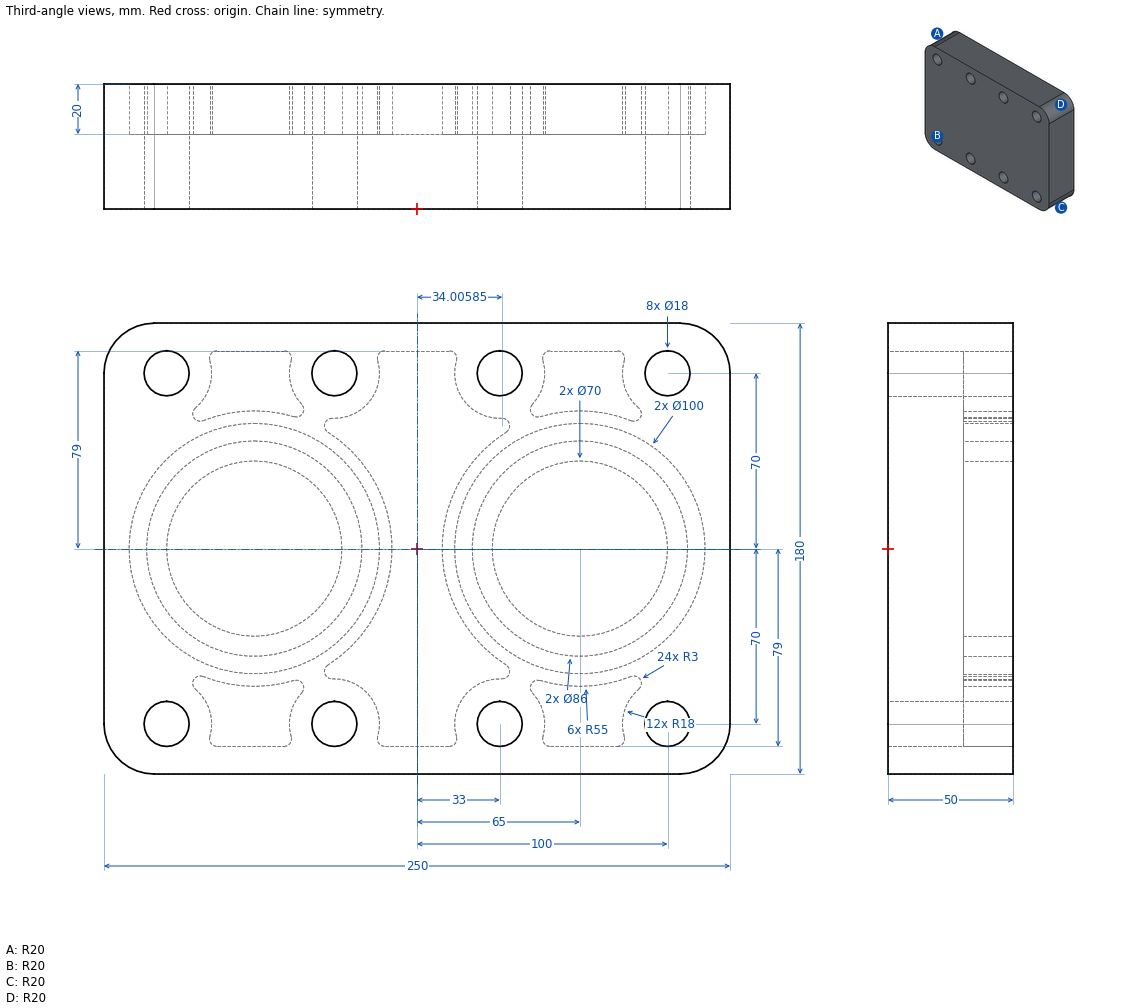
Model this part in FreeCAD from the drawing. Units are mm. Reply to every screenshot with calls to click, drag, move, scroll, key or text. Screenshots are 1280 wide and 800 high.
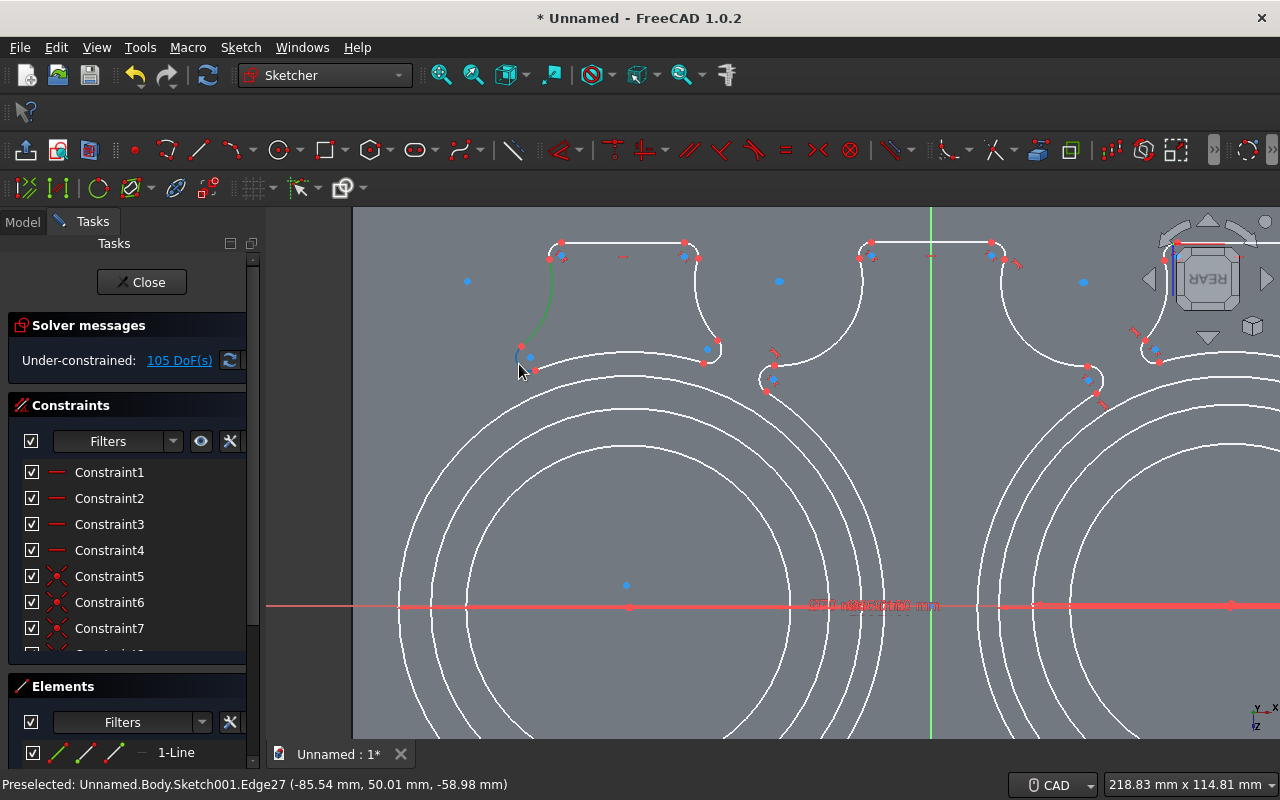
click(518, 365)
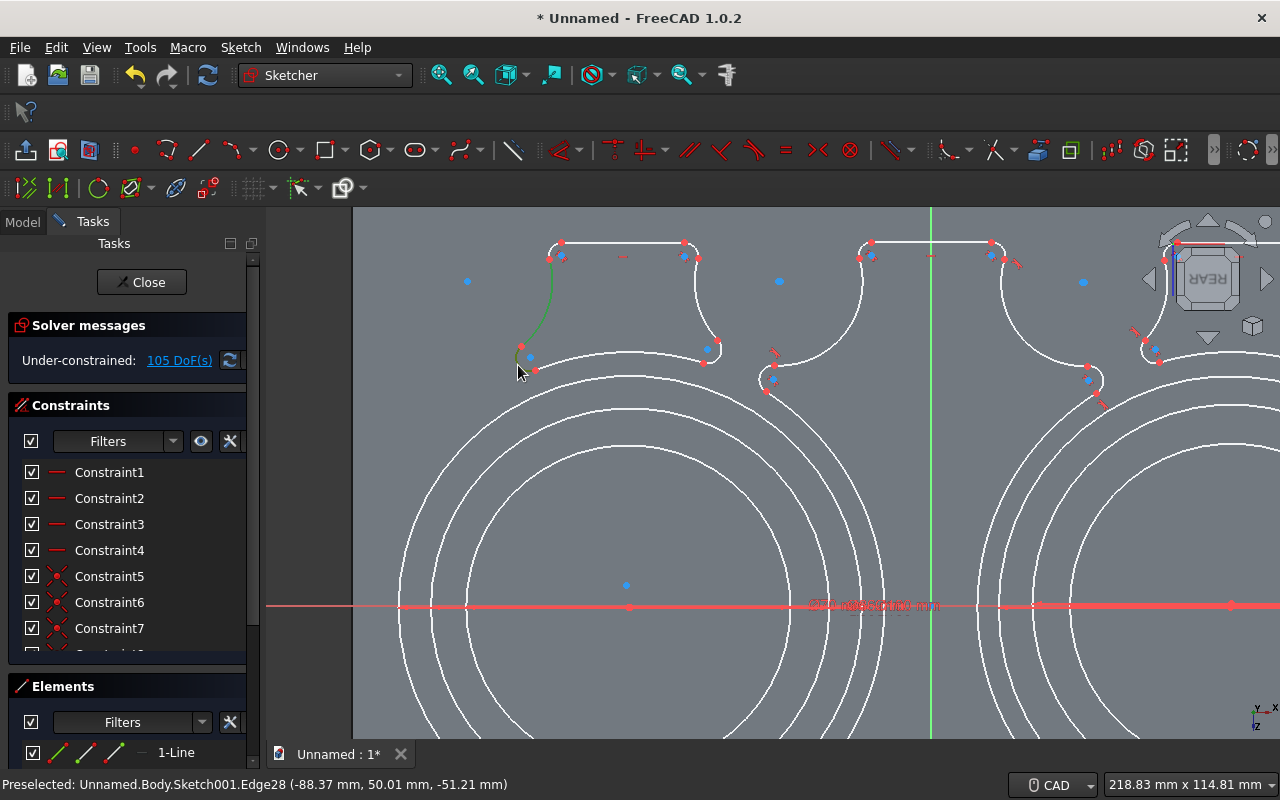
click(754, 150)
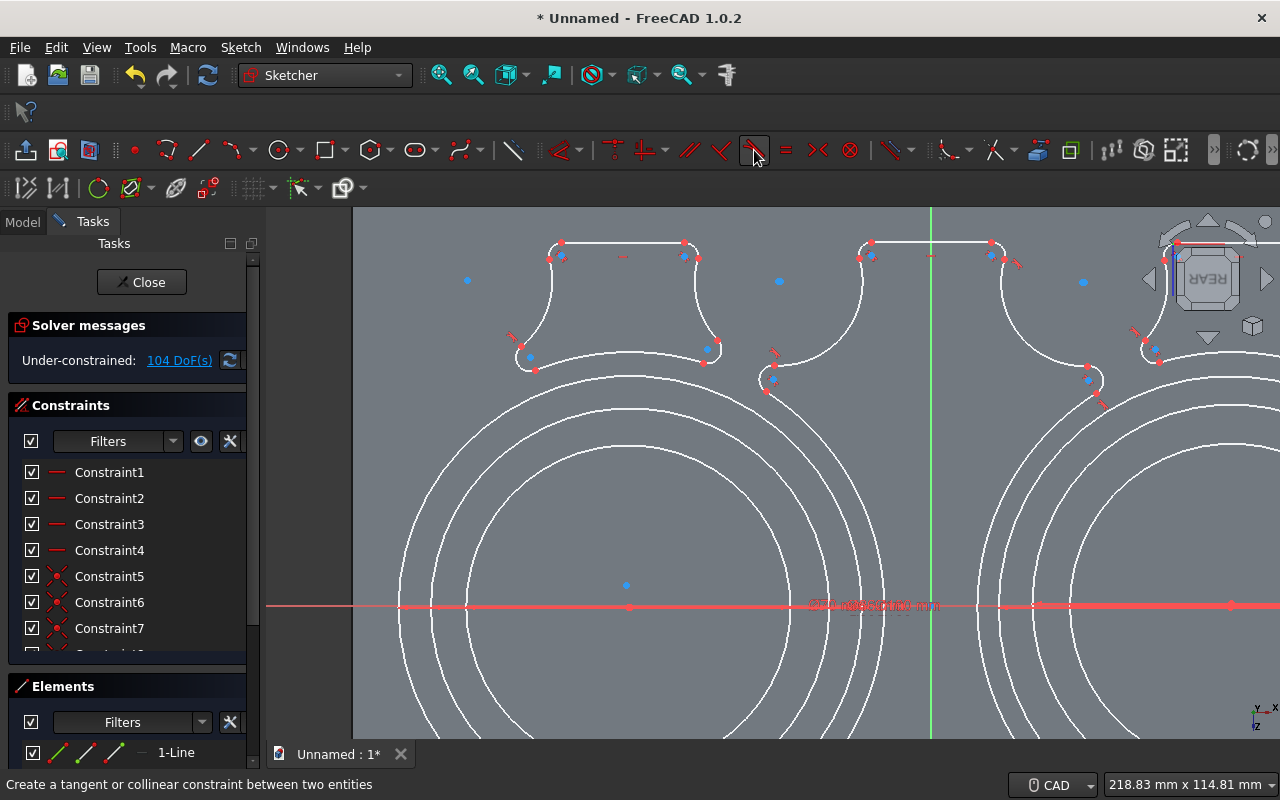
click(516, 357)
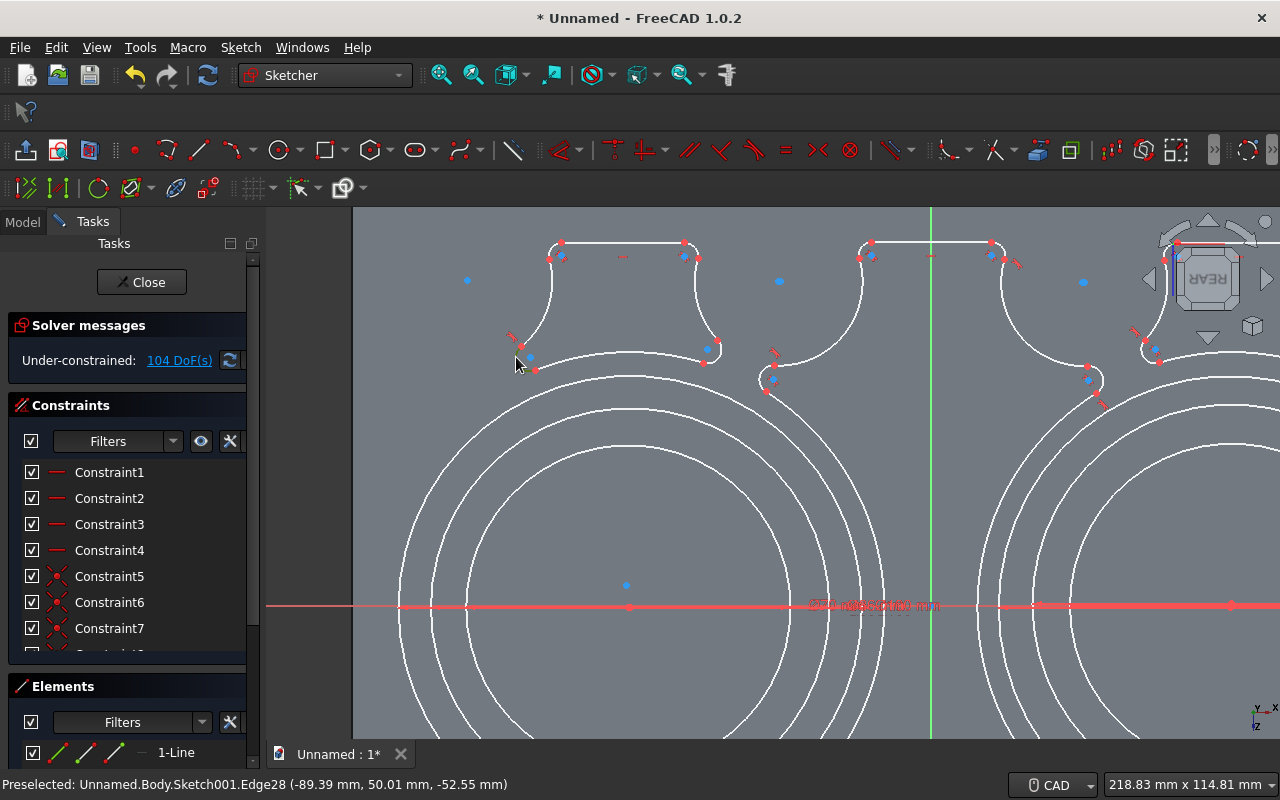
click(653, 353)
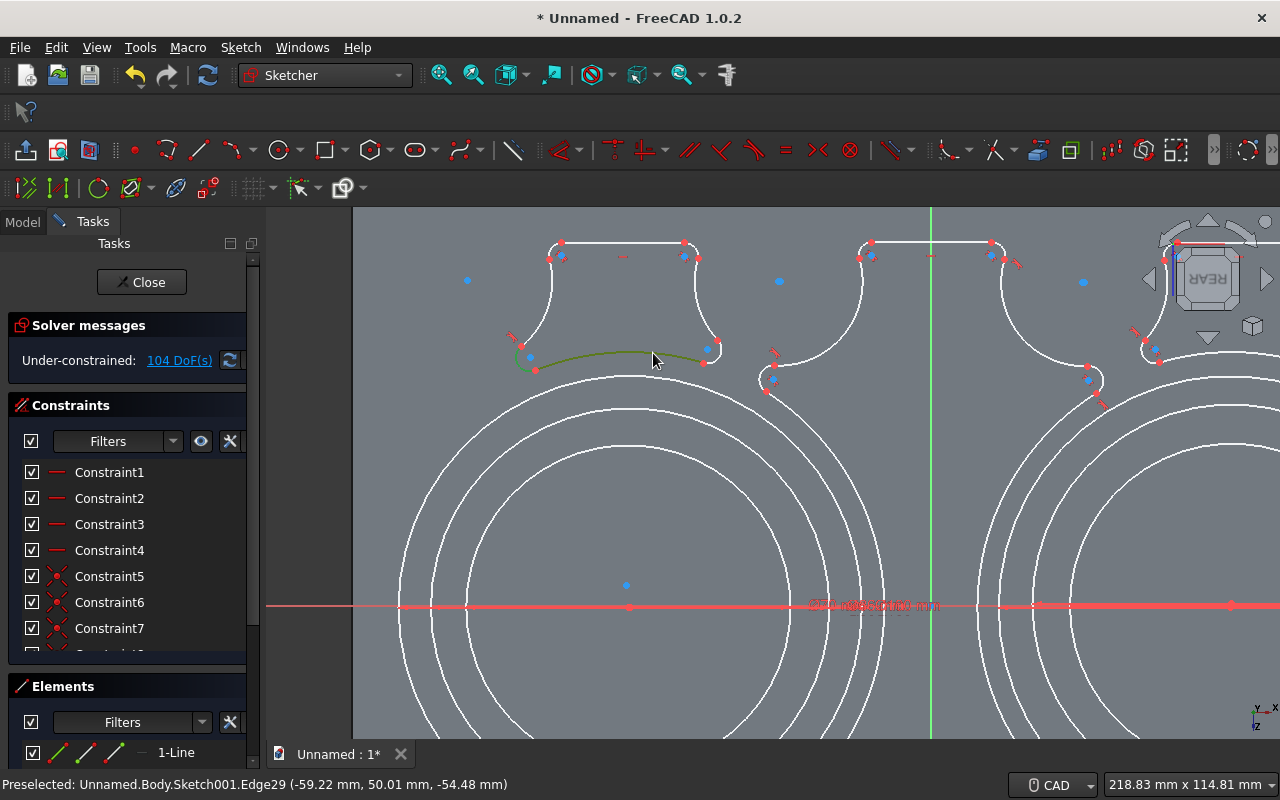
click(754, 150)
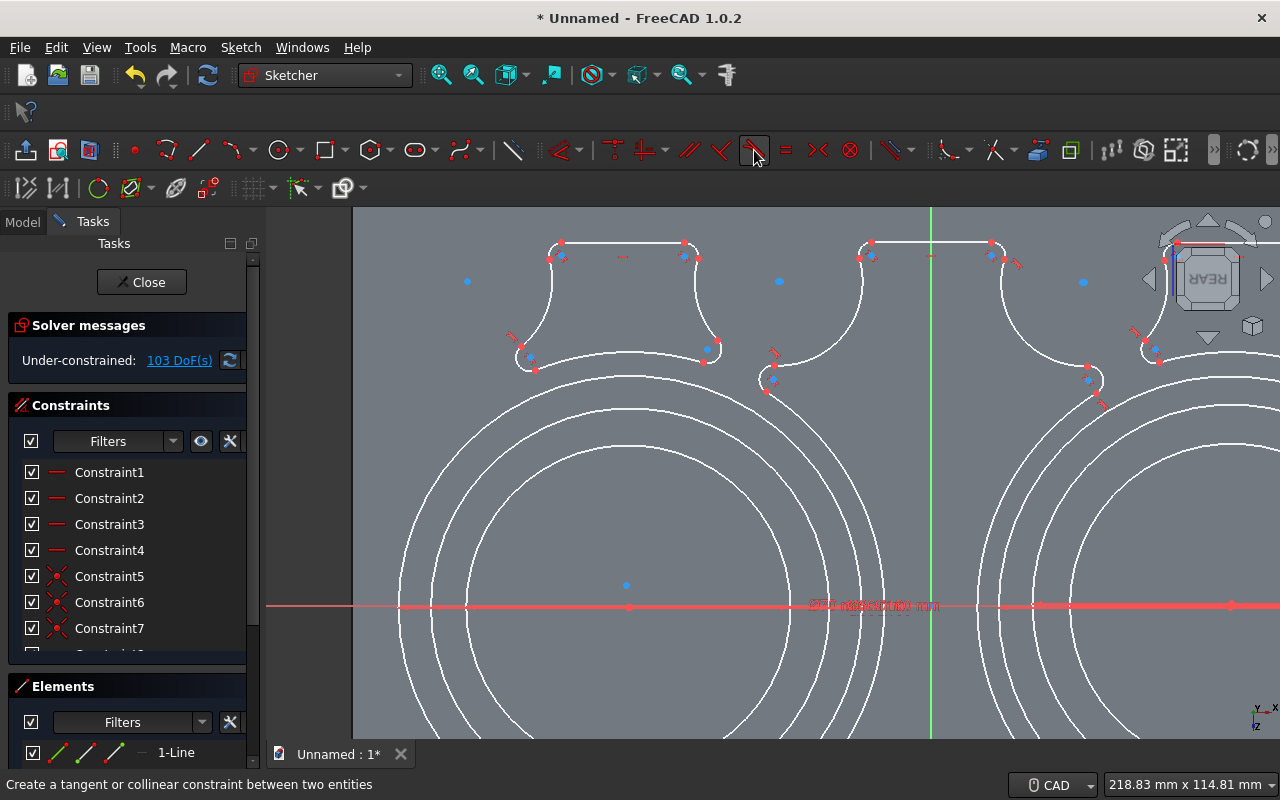
click(653, 353)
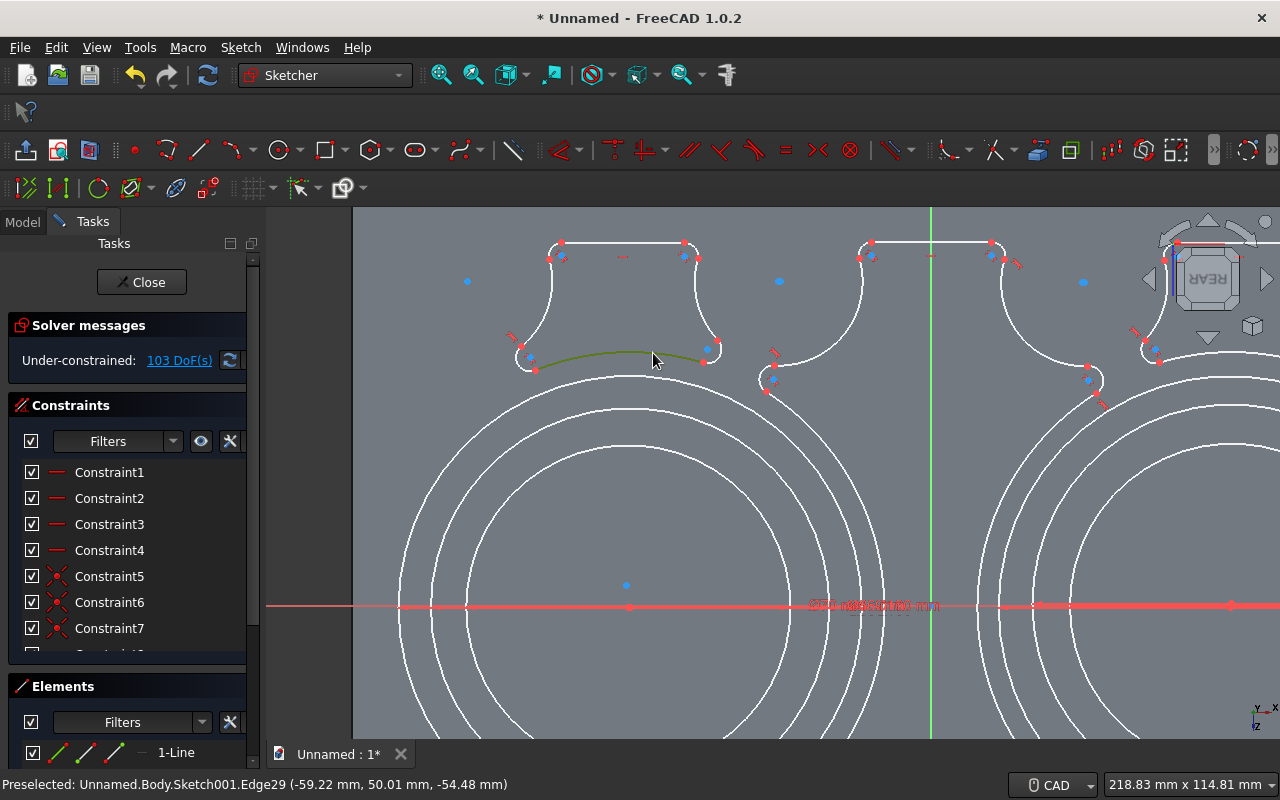
scroll(714, 362, up, 2)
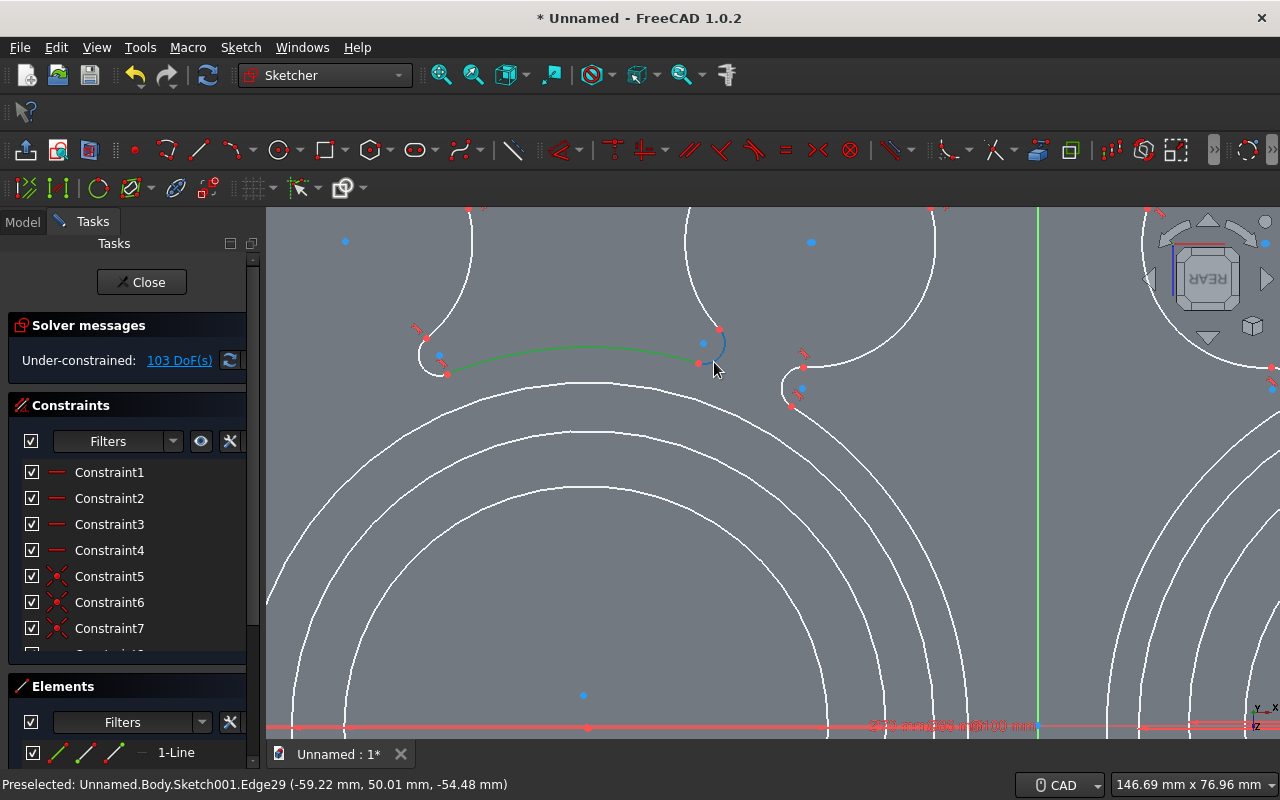
click(714, 361)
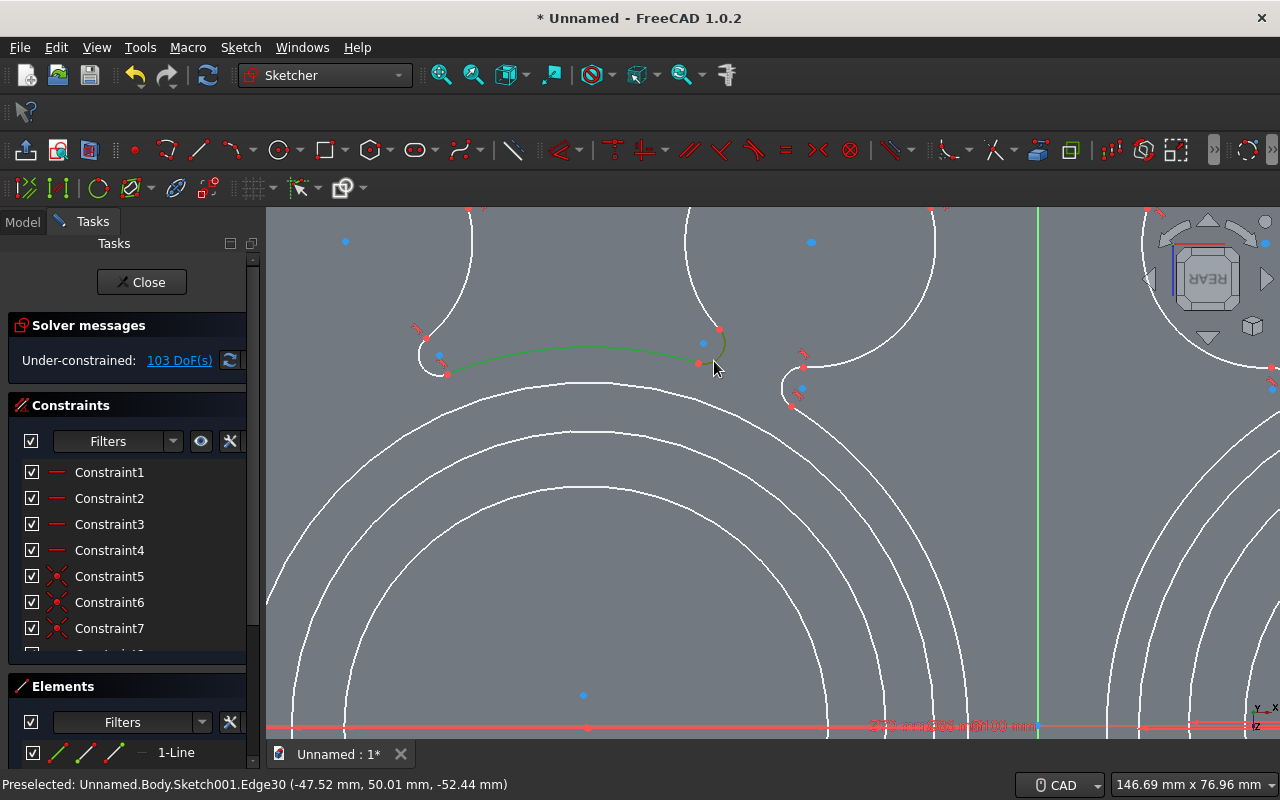
click(754, 150)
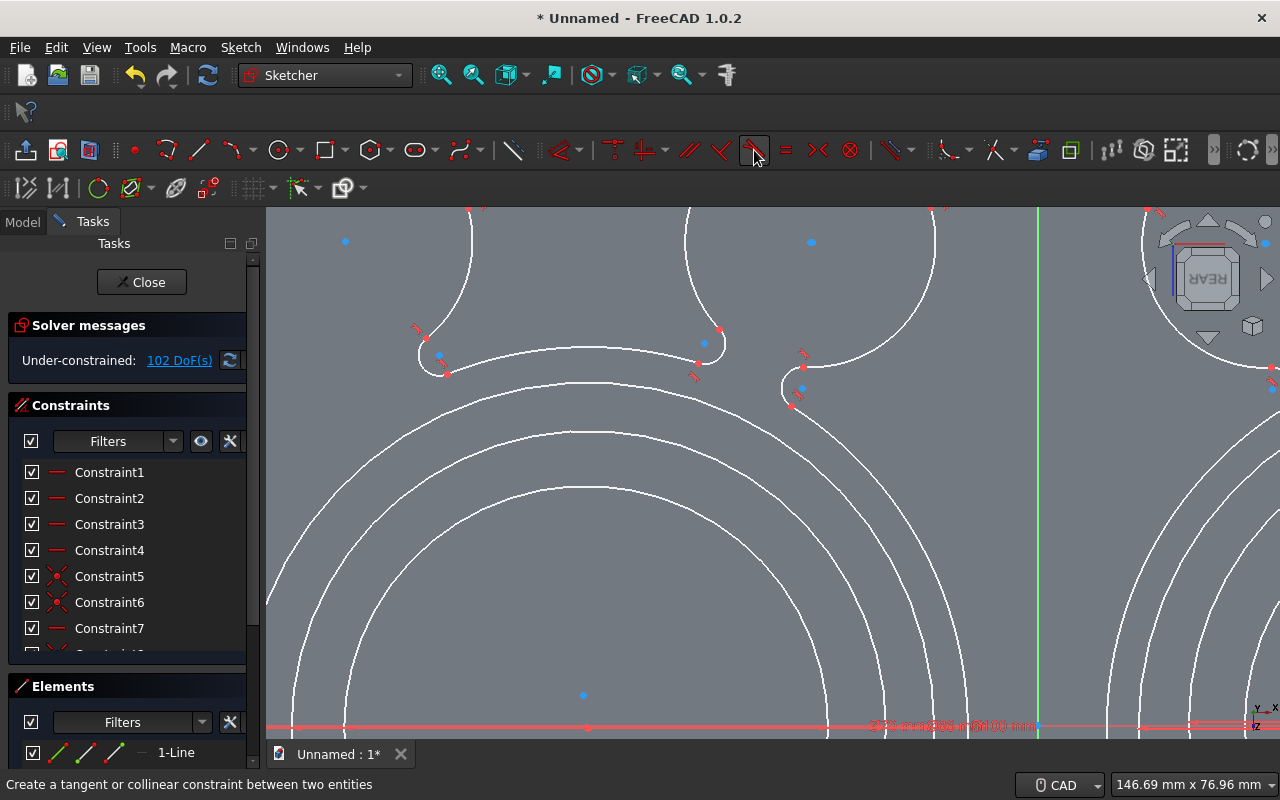
click(715, 362)